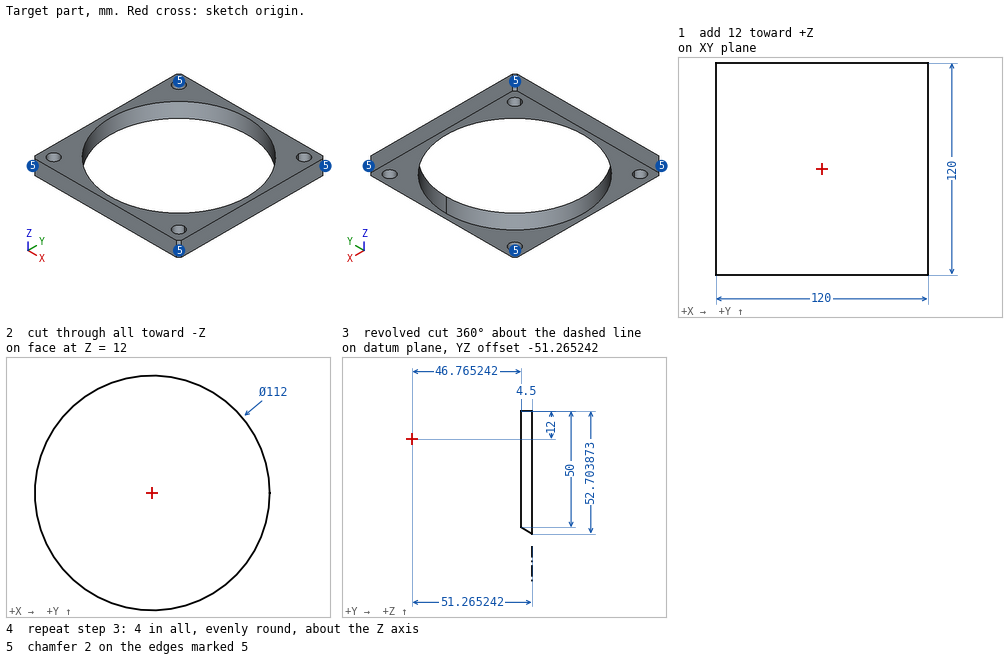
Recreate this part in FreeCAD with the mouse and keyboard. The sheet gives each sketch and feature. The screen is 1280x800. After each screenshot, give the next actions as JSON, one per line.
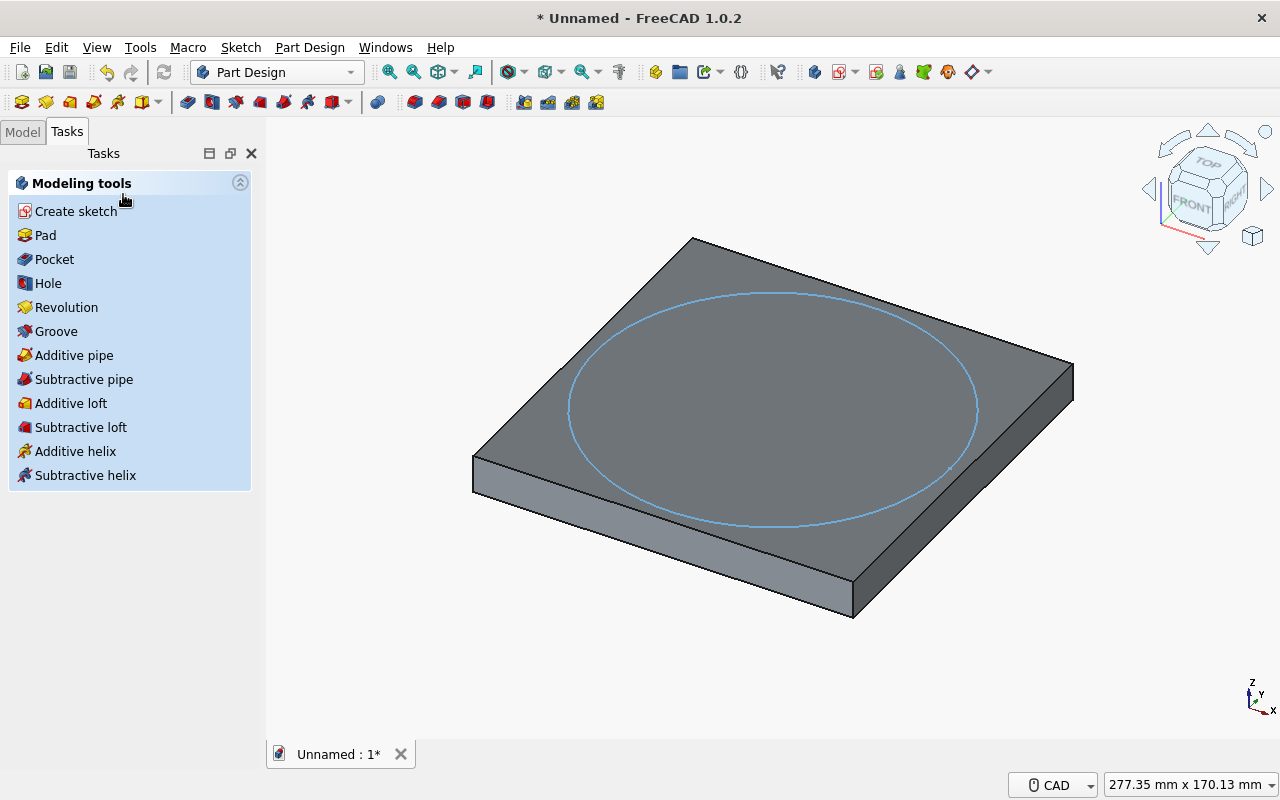
{"action": "left_click", "coordinate": [188, 102]}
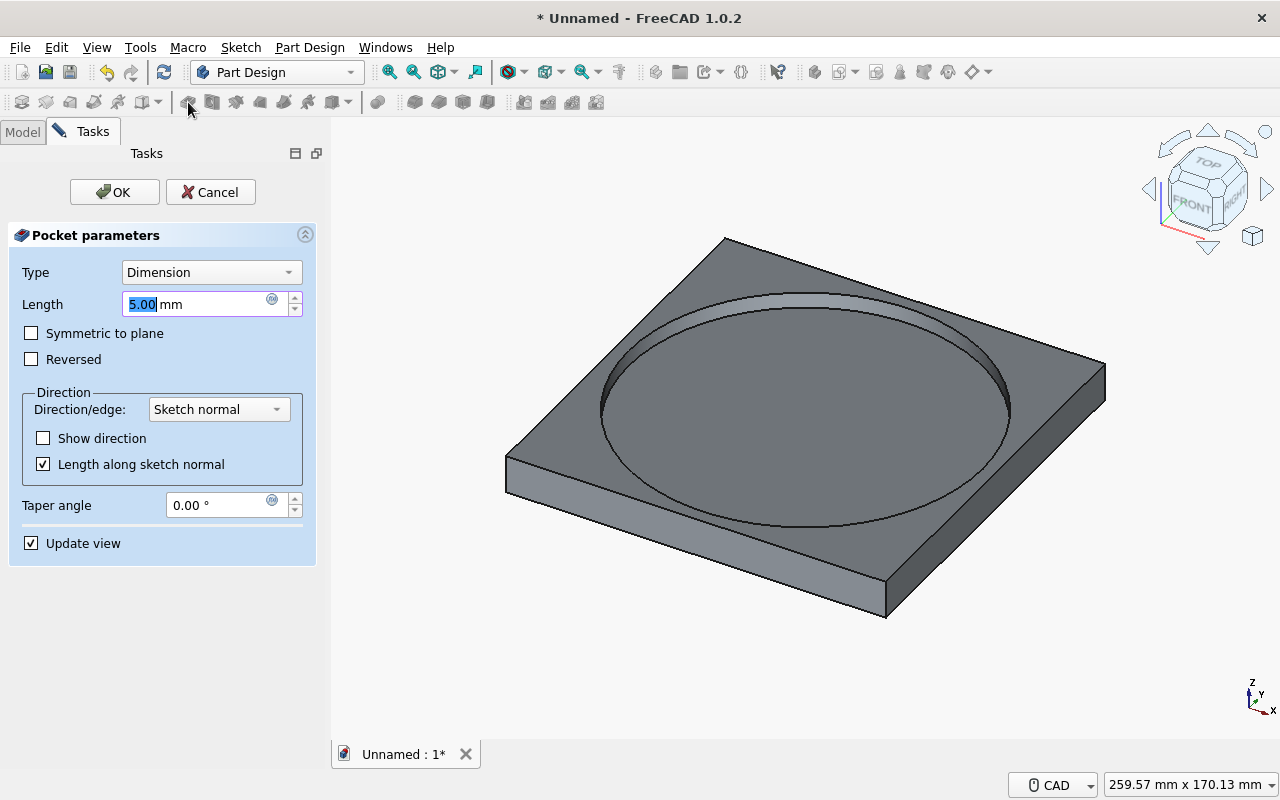
{"action": "left_click", "coordinate": [212, 272]}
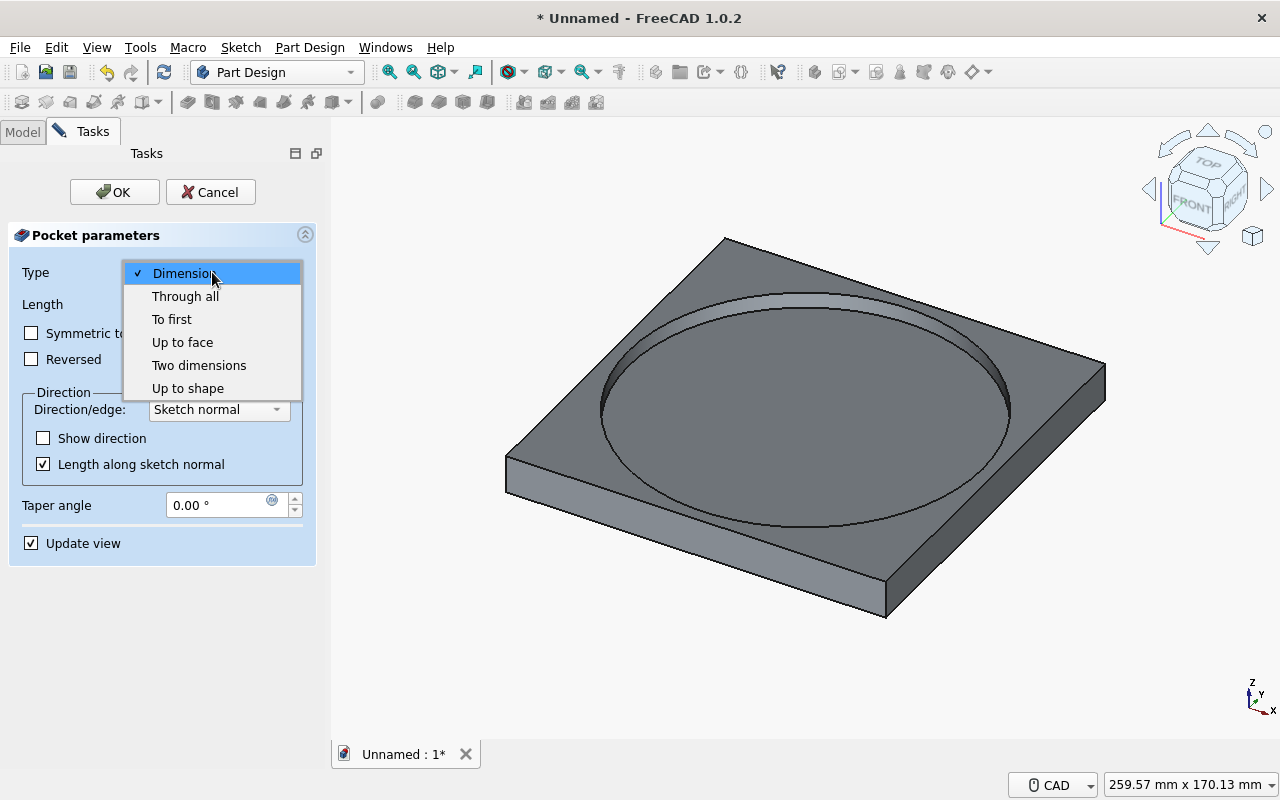
{"action": "left_click", "coordinate": [212, 296]}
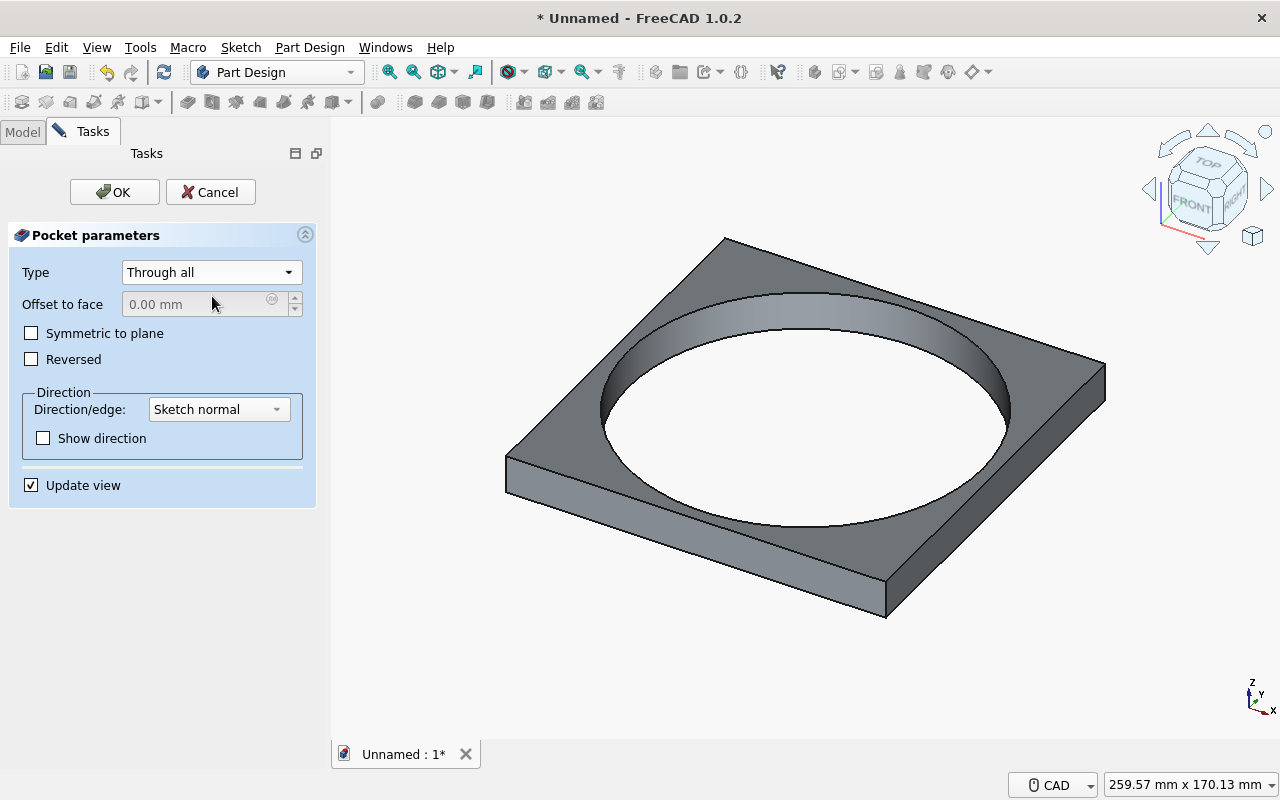
{"action": "left_click", "coordinate": [115, 192]}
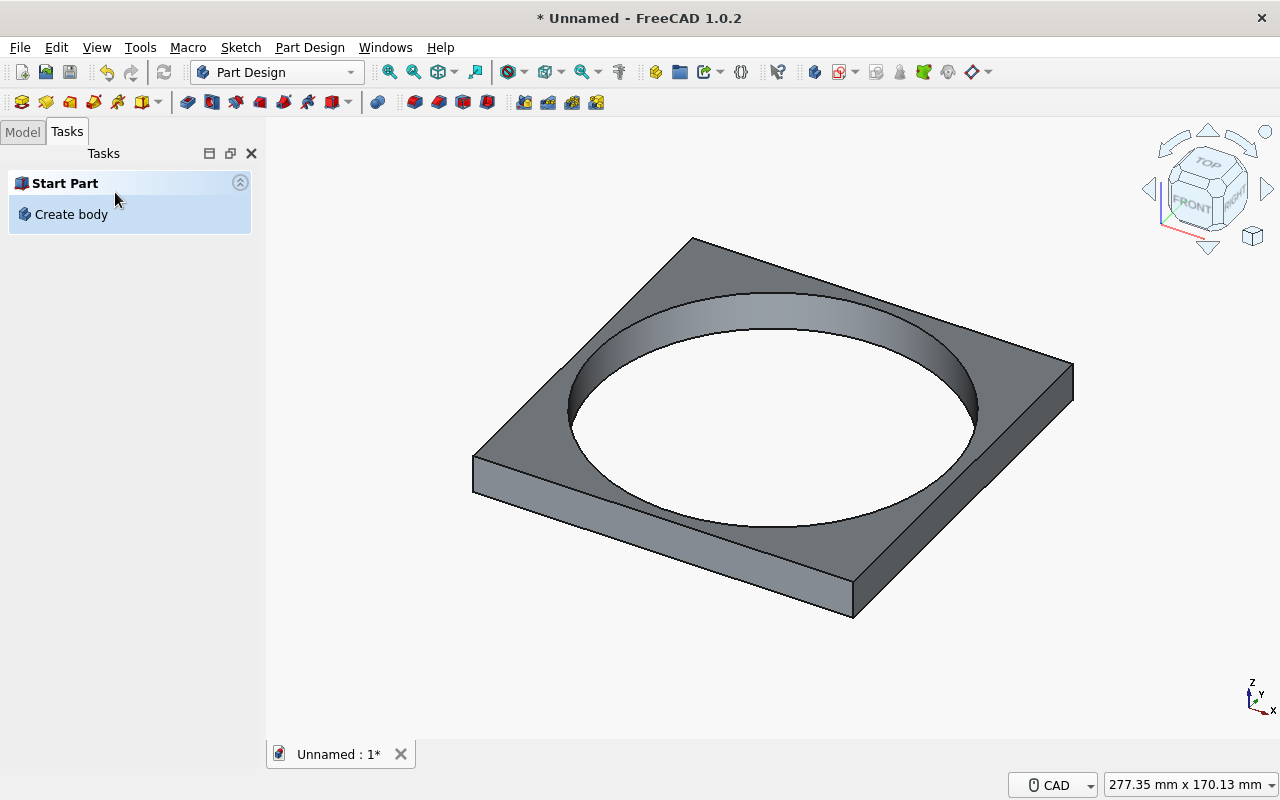
{"action": "left_click", "coordinate": [23, 131]}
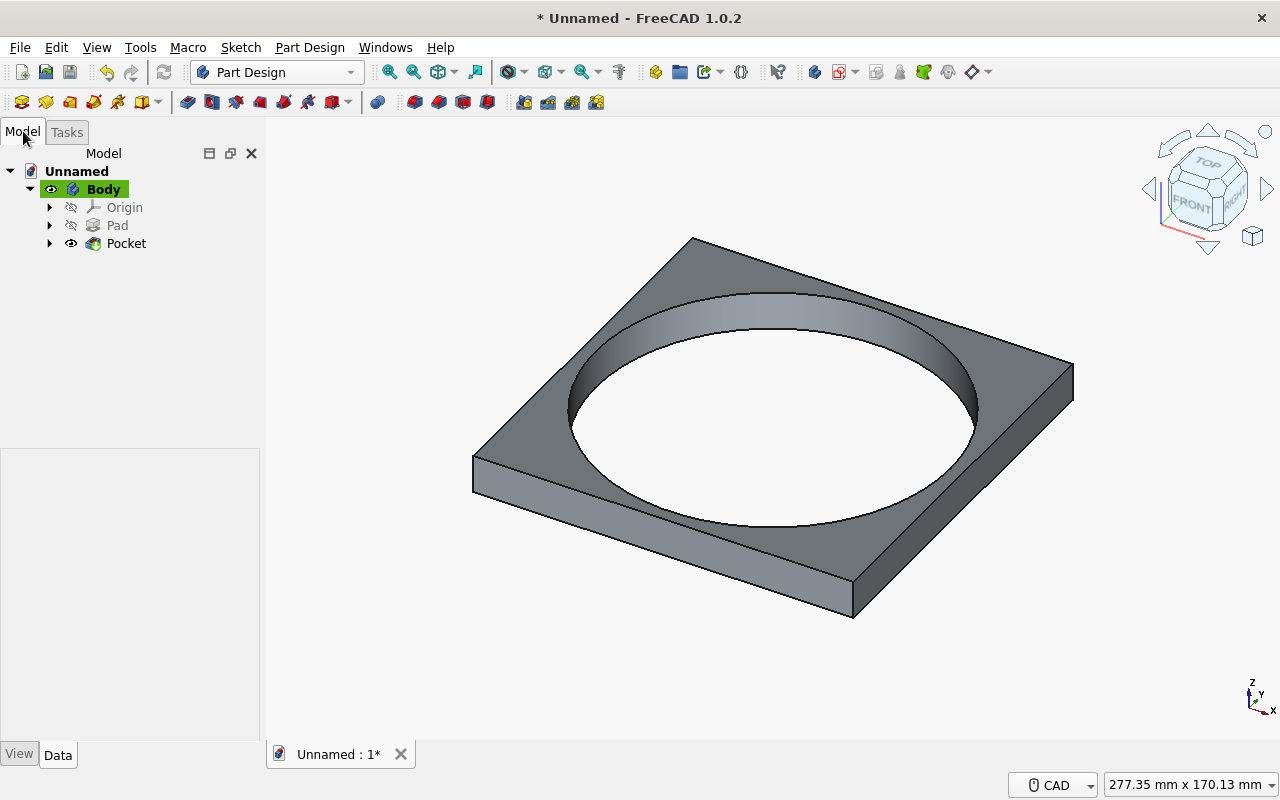
{"action": "left_click", "coordinate": [50, 207]}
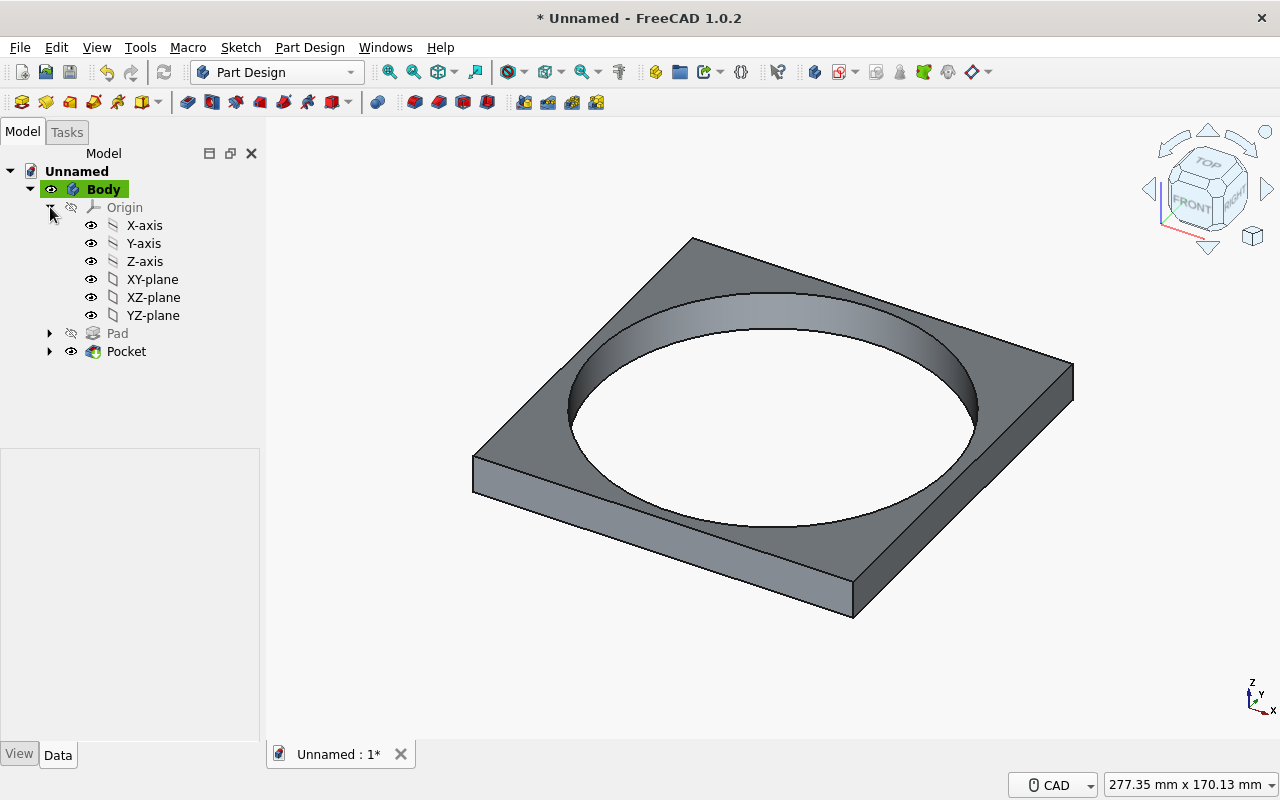
{"action": "left_click", "coordinate": [136, 315]}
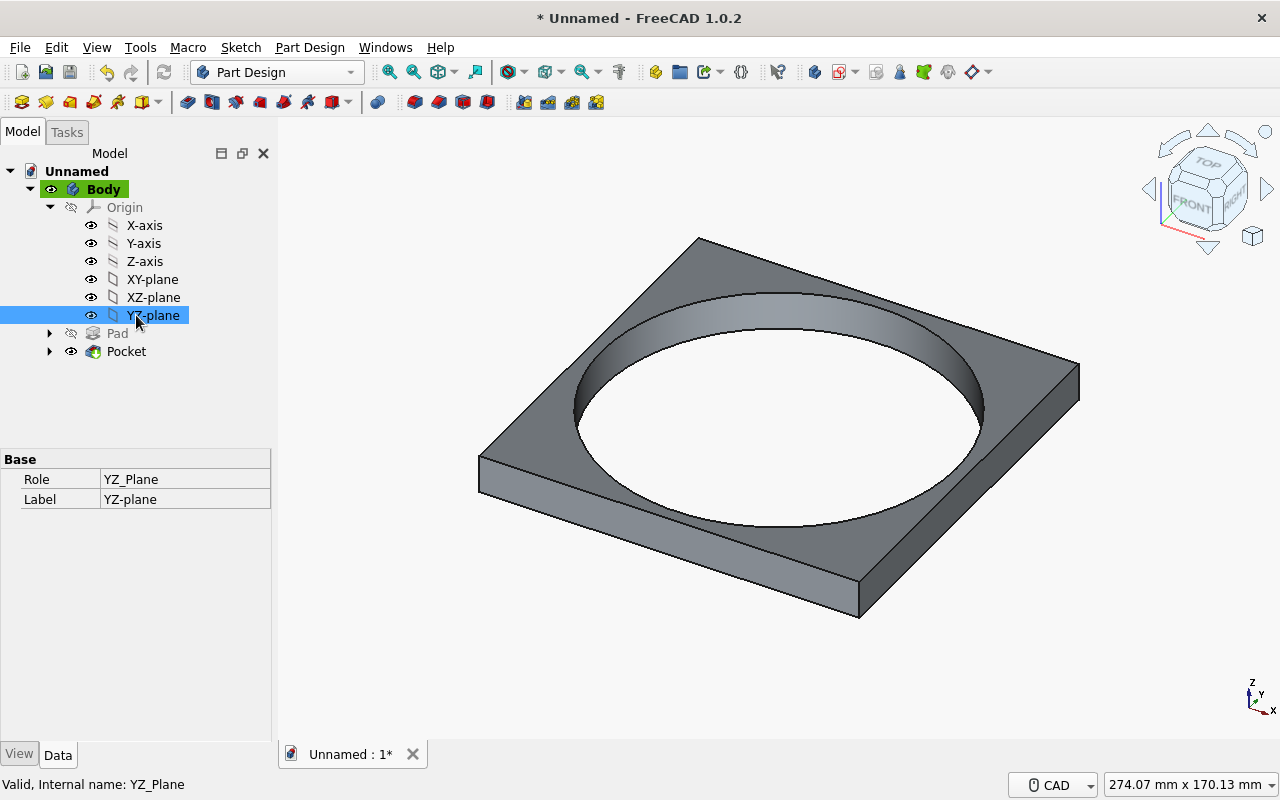
{"action": "left_click", "coordinate": [972, 72]}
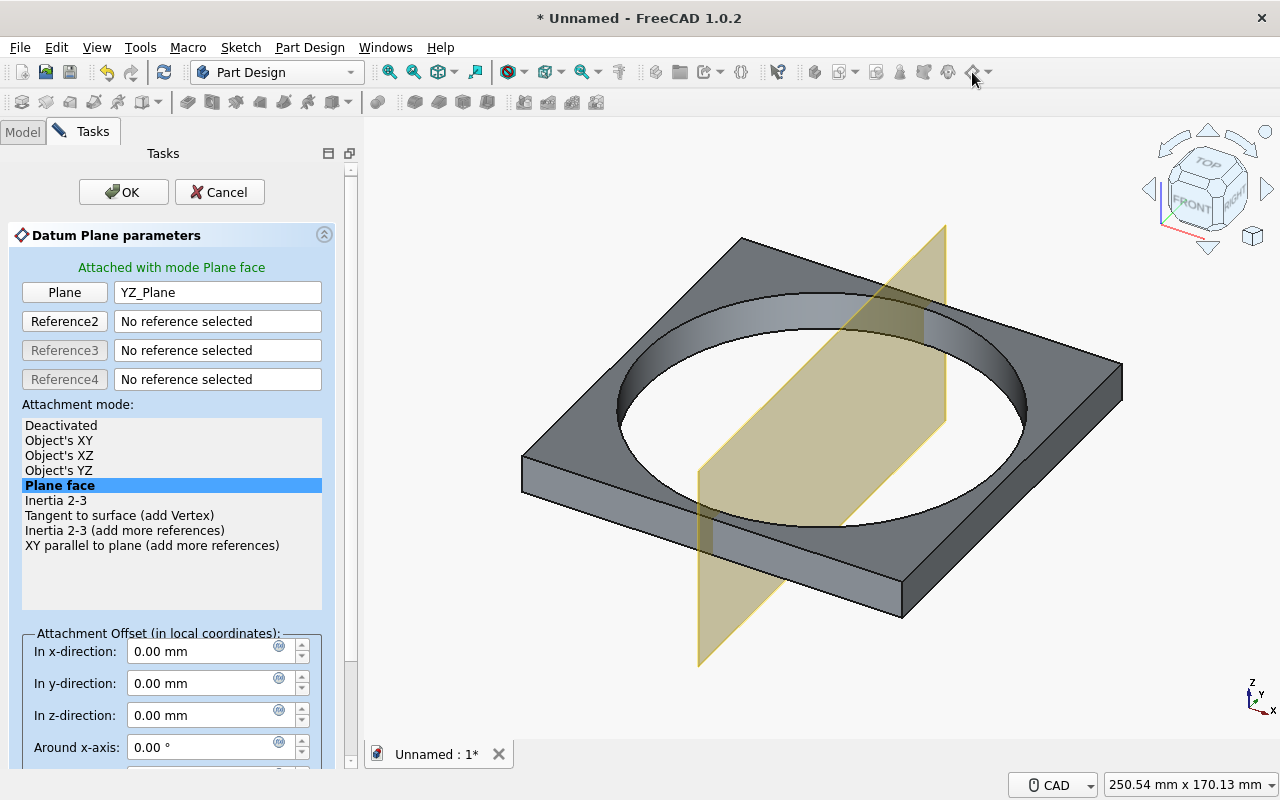
{"action": "triple_click", "coordinate": [210, 715]}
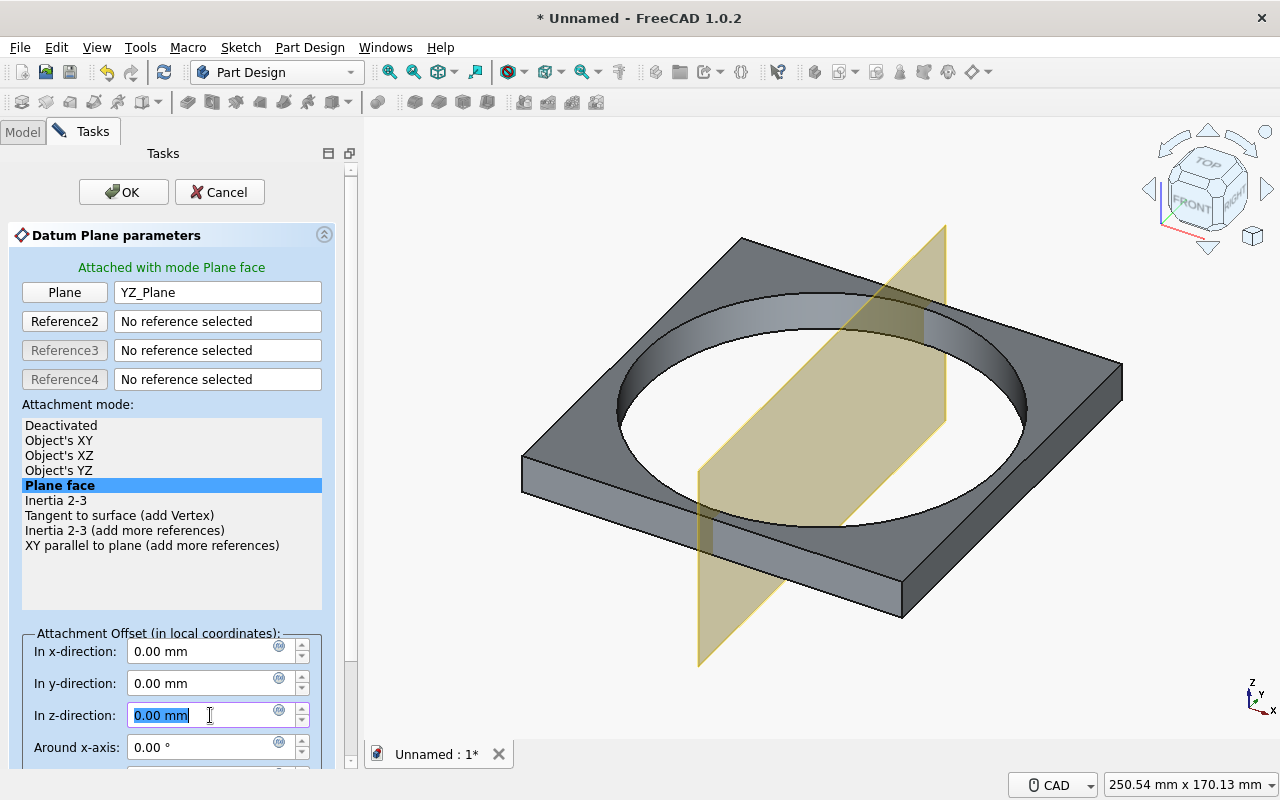
{"action": "type", "text": "-51.265242"}
{"action": "key", "text": "Tab"}